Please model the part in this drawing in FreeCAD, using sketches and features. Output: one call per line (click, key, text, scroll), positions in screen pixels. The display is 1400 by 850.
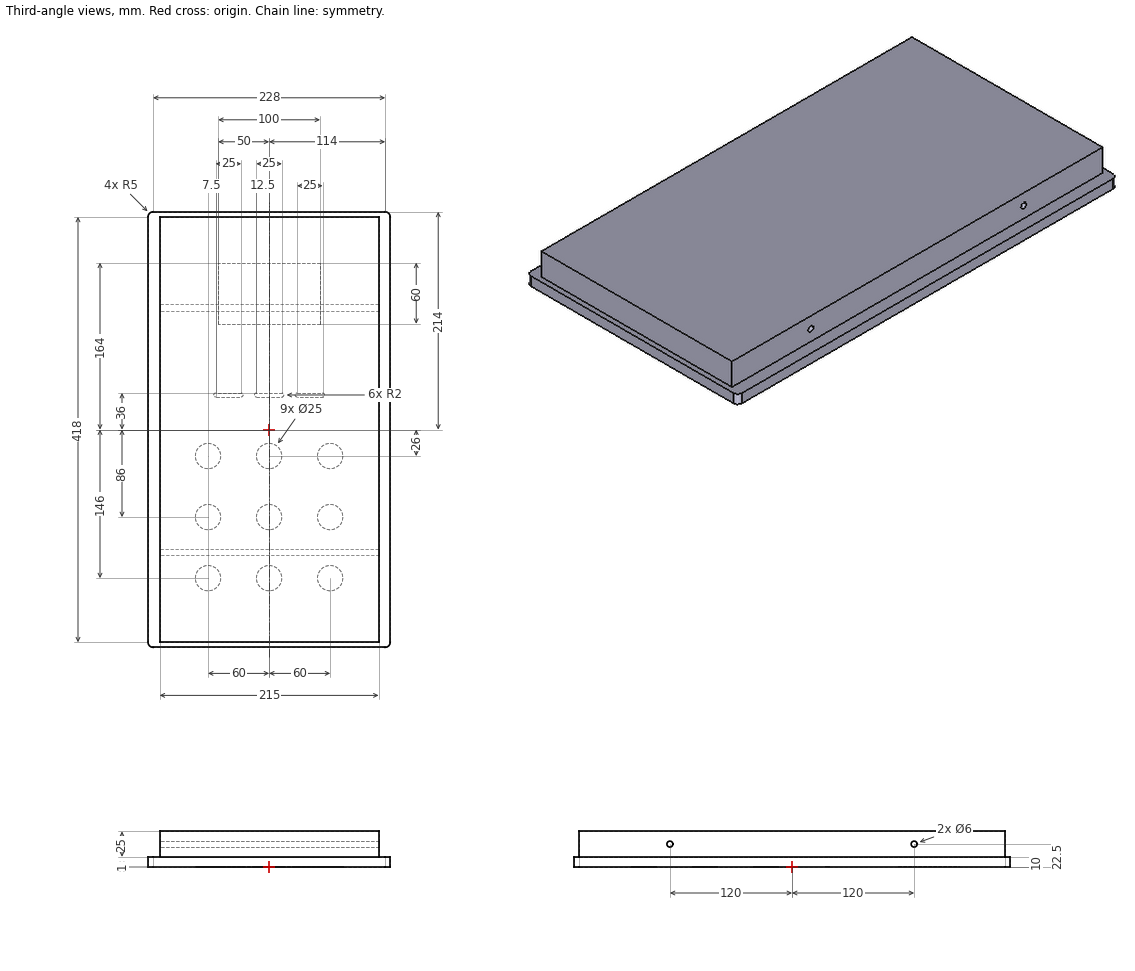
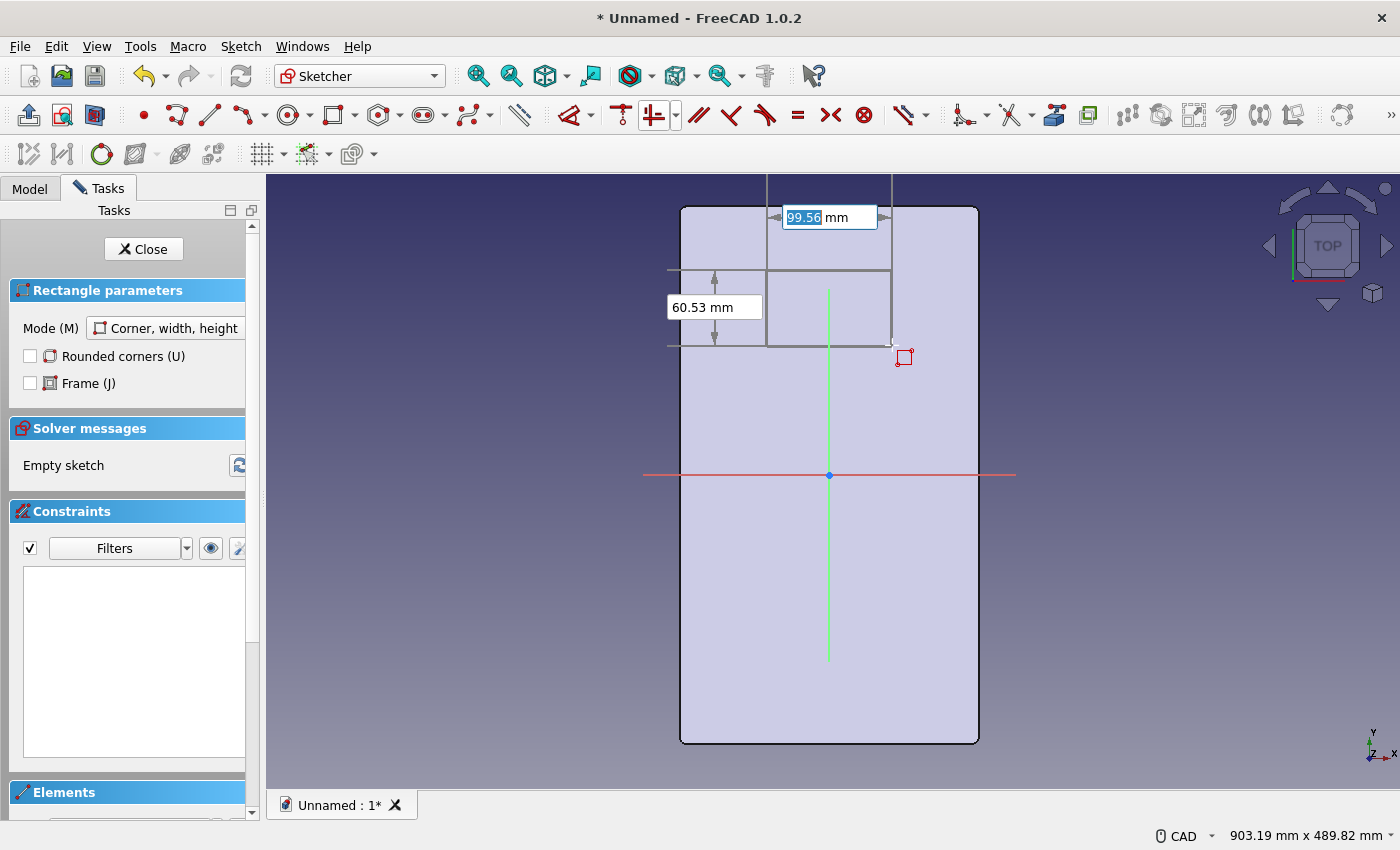
text(100)
key(Tab)
text(60)
key(Return)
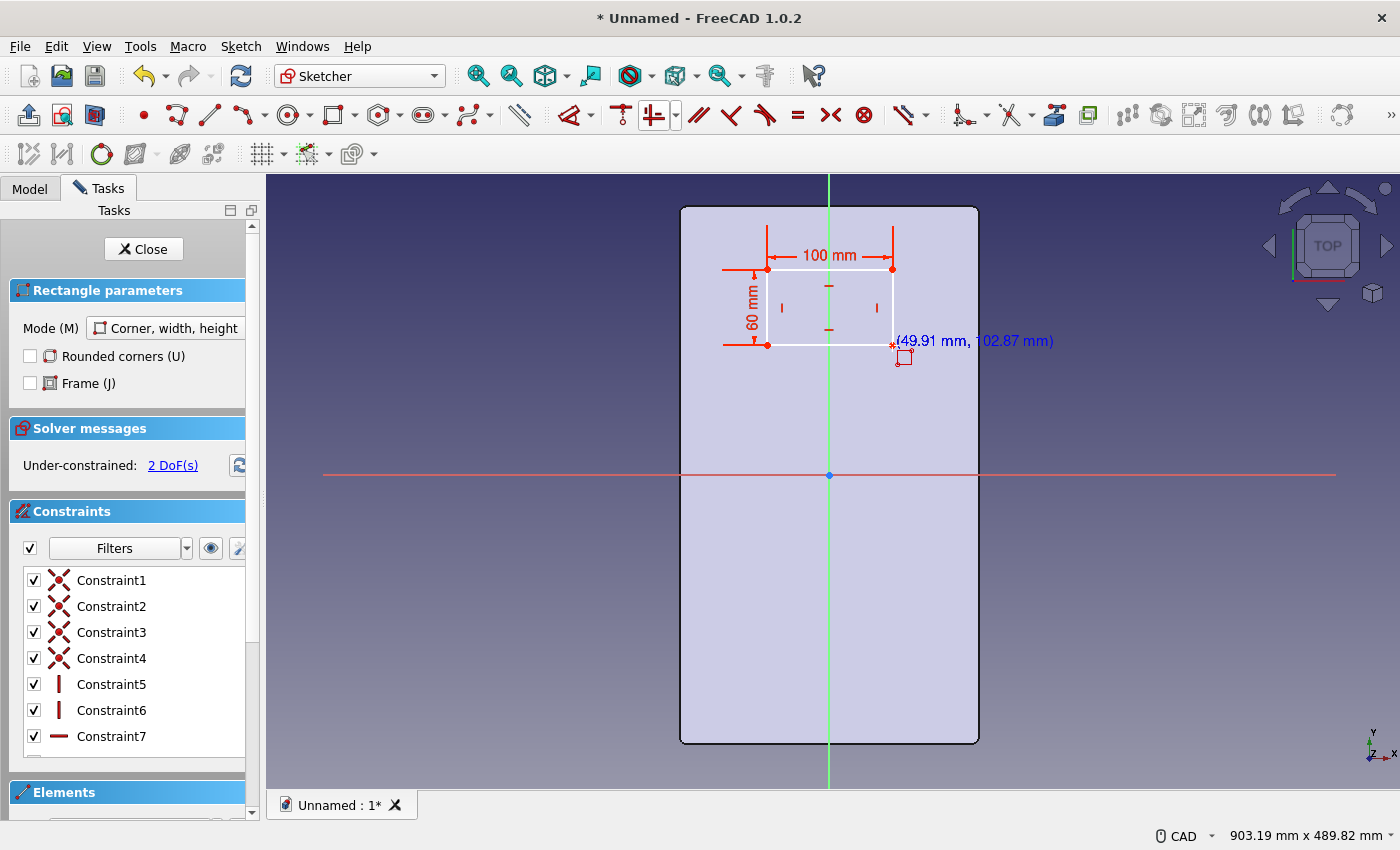
key(g)
key(s)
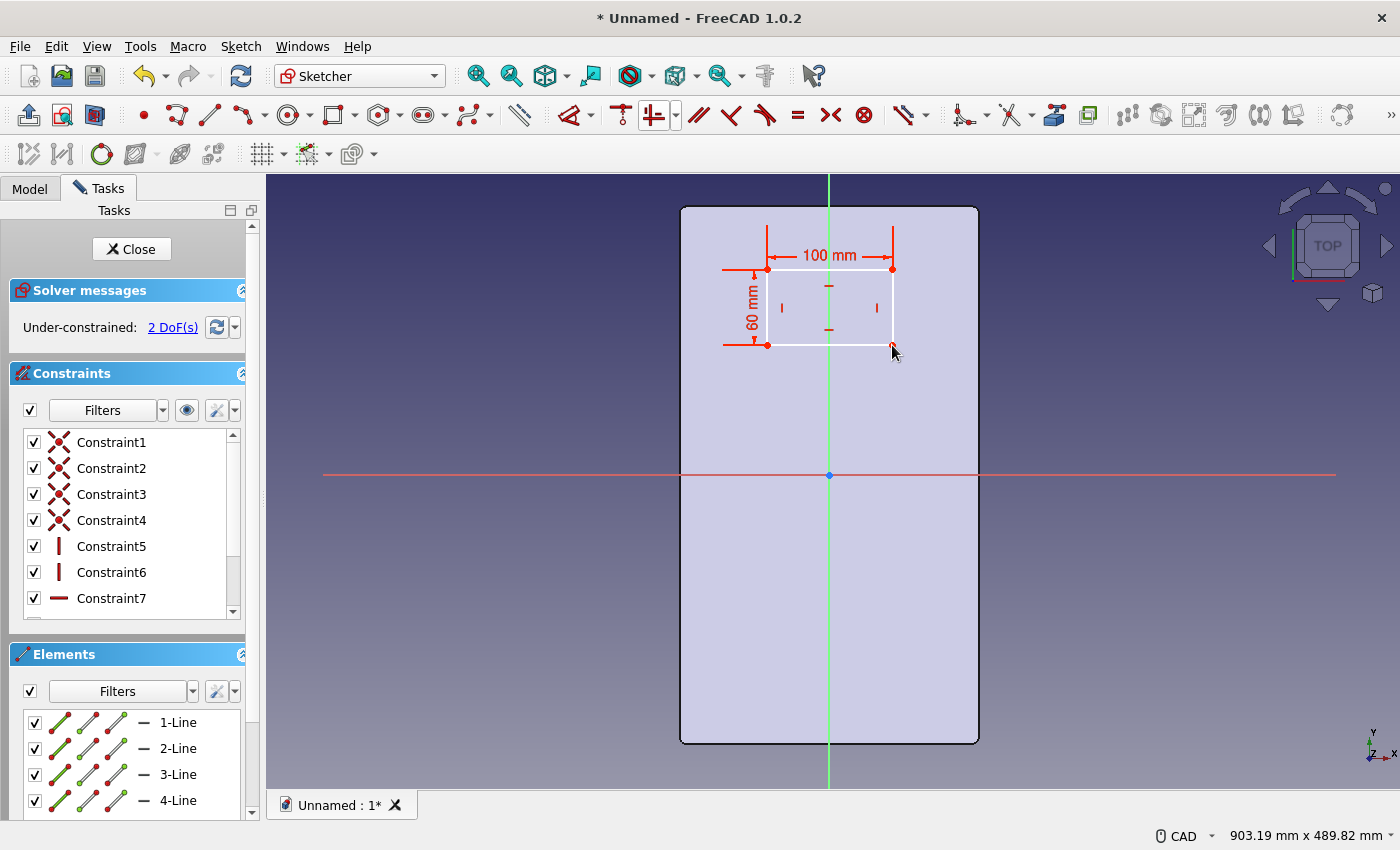
scroll(814, 432, up, 12)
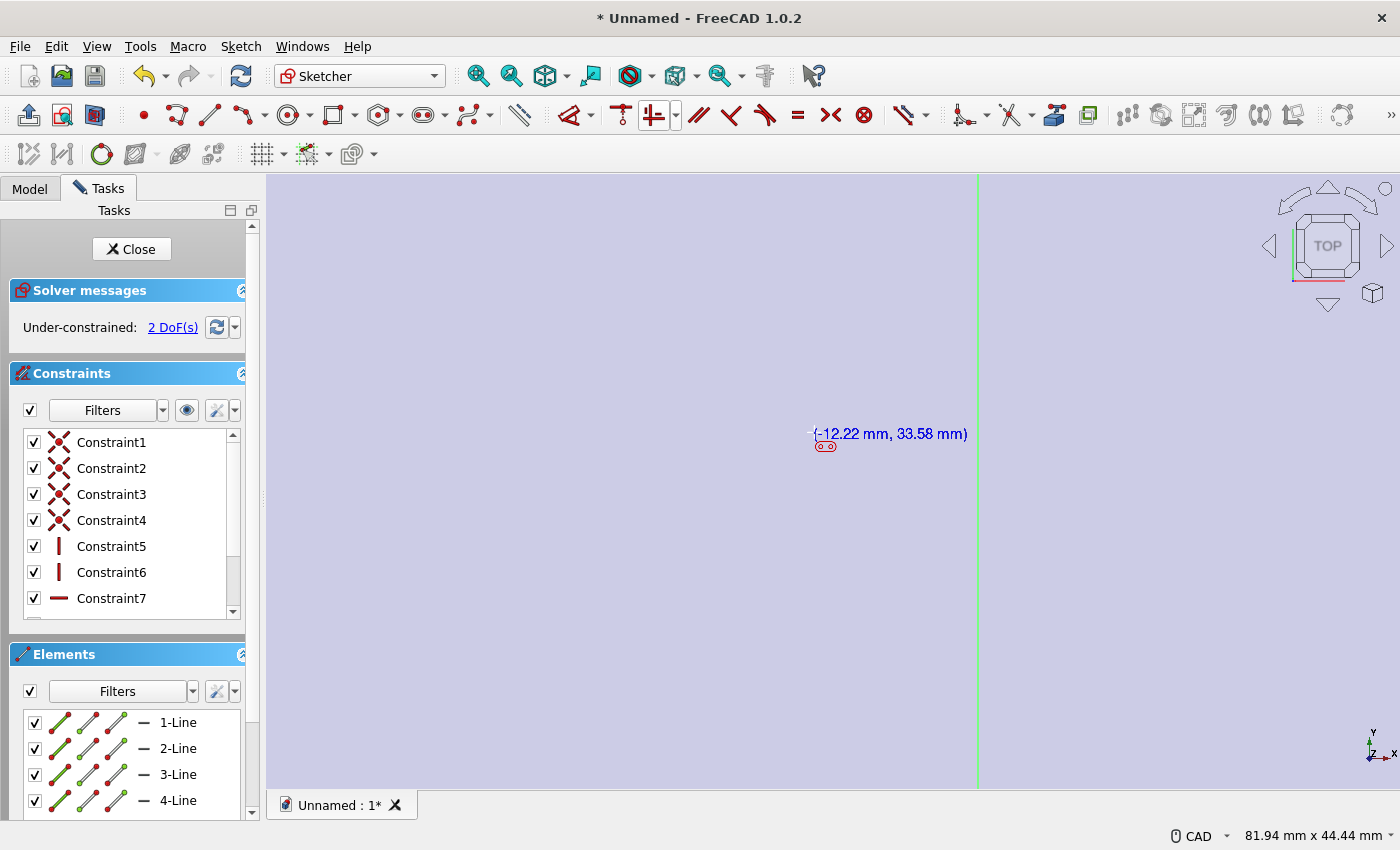
scroll(743, 443, down, 12)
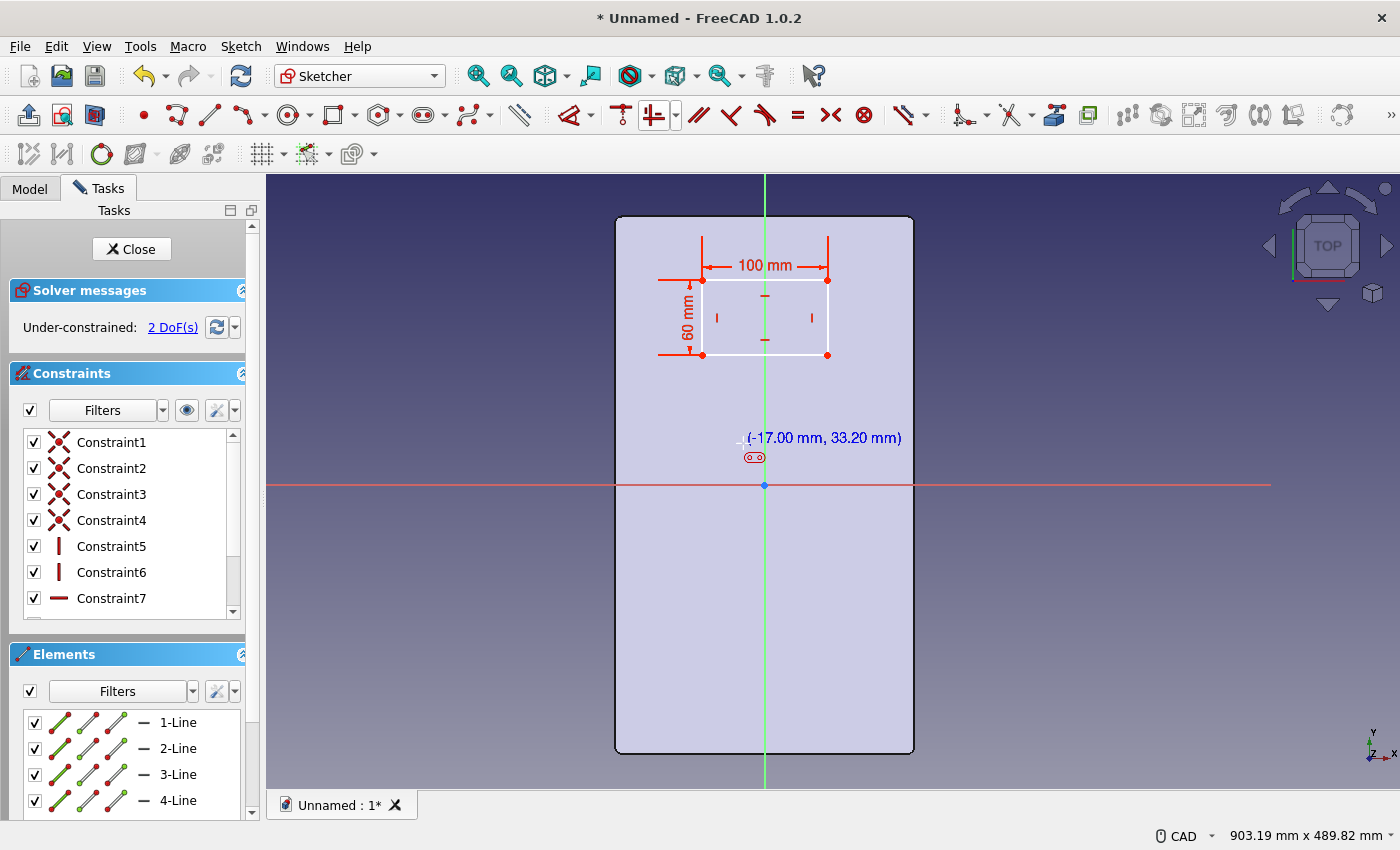
click(749, 442)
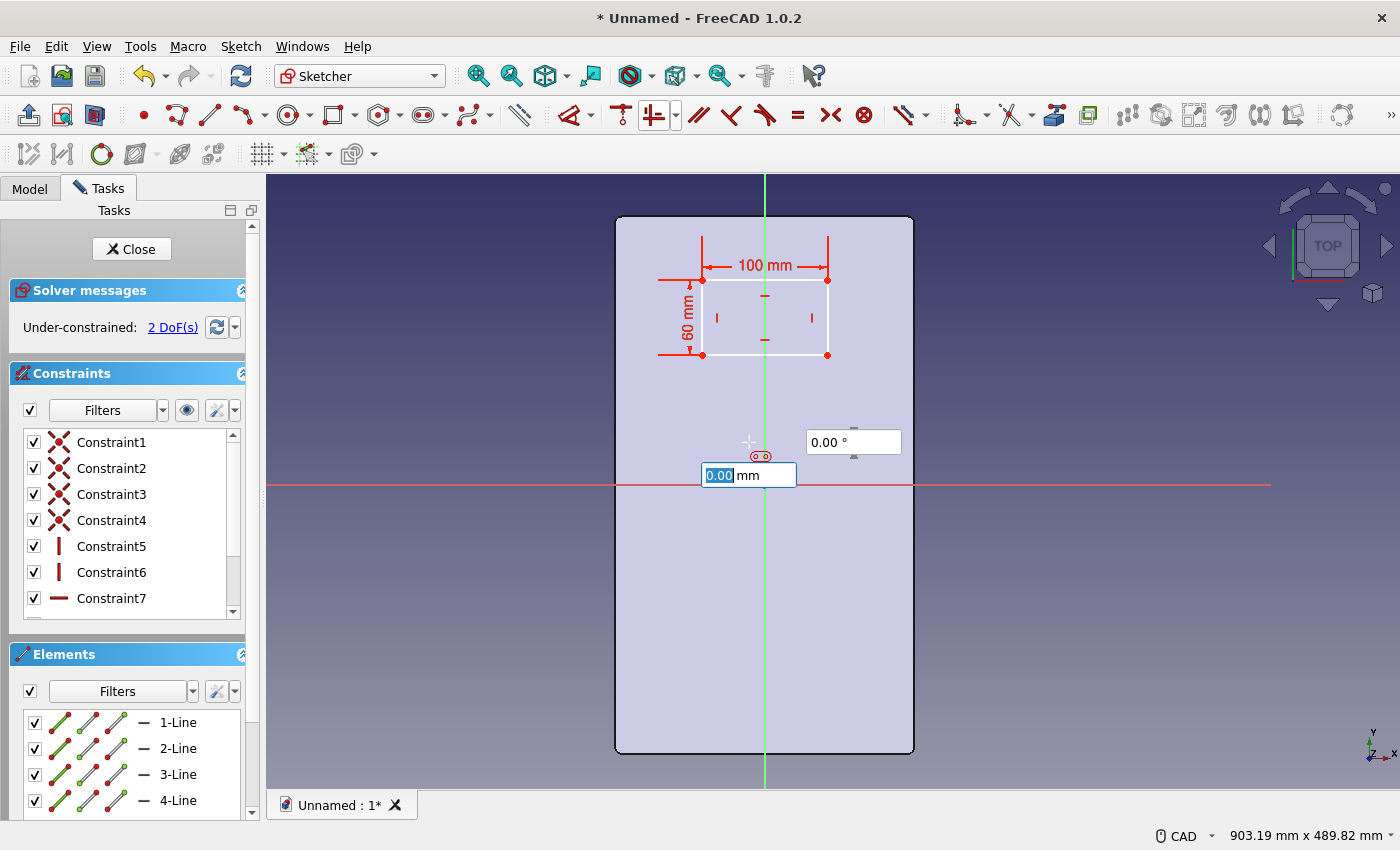
click(780, 442)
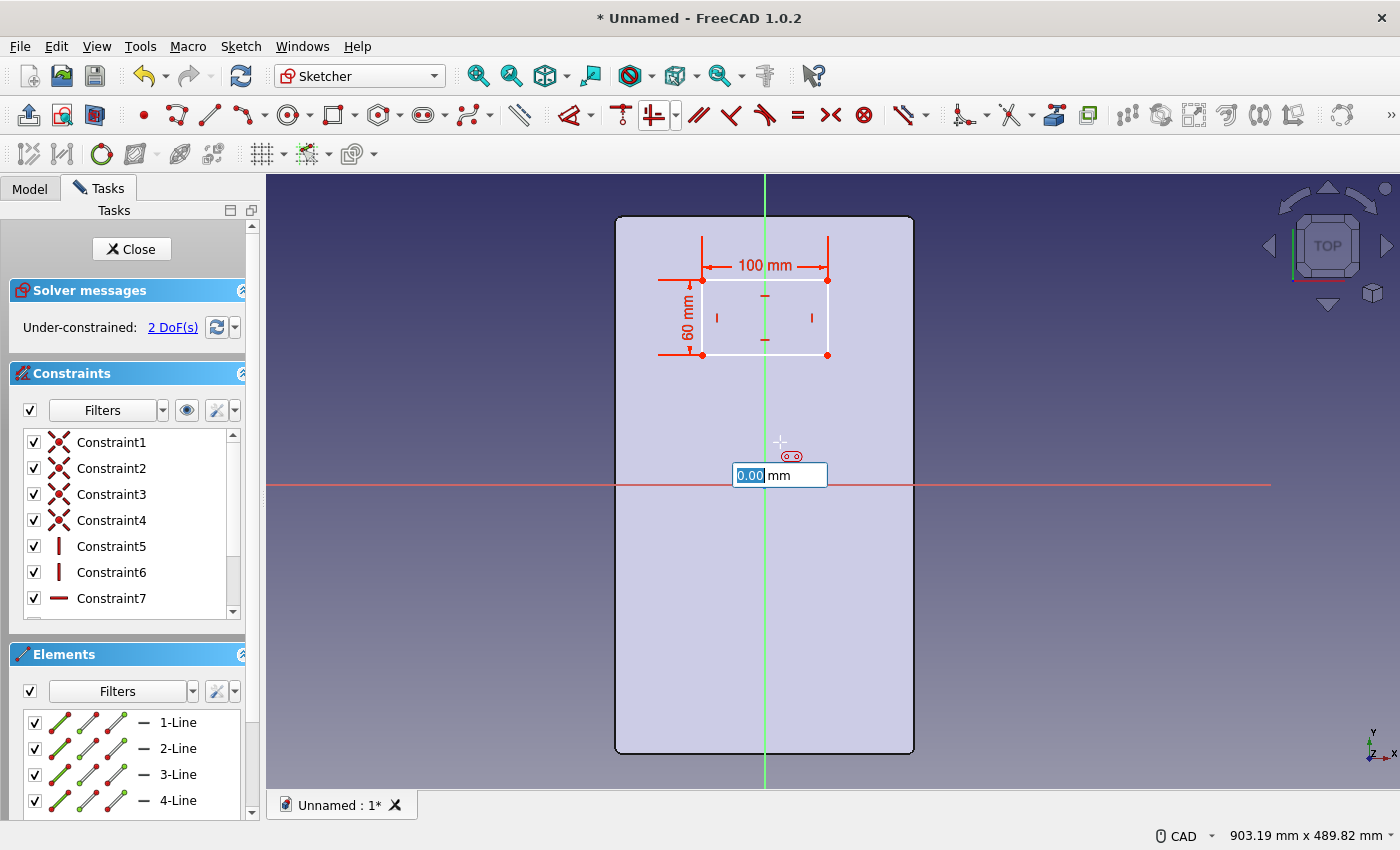
scroll(760, 440, up, 10)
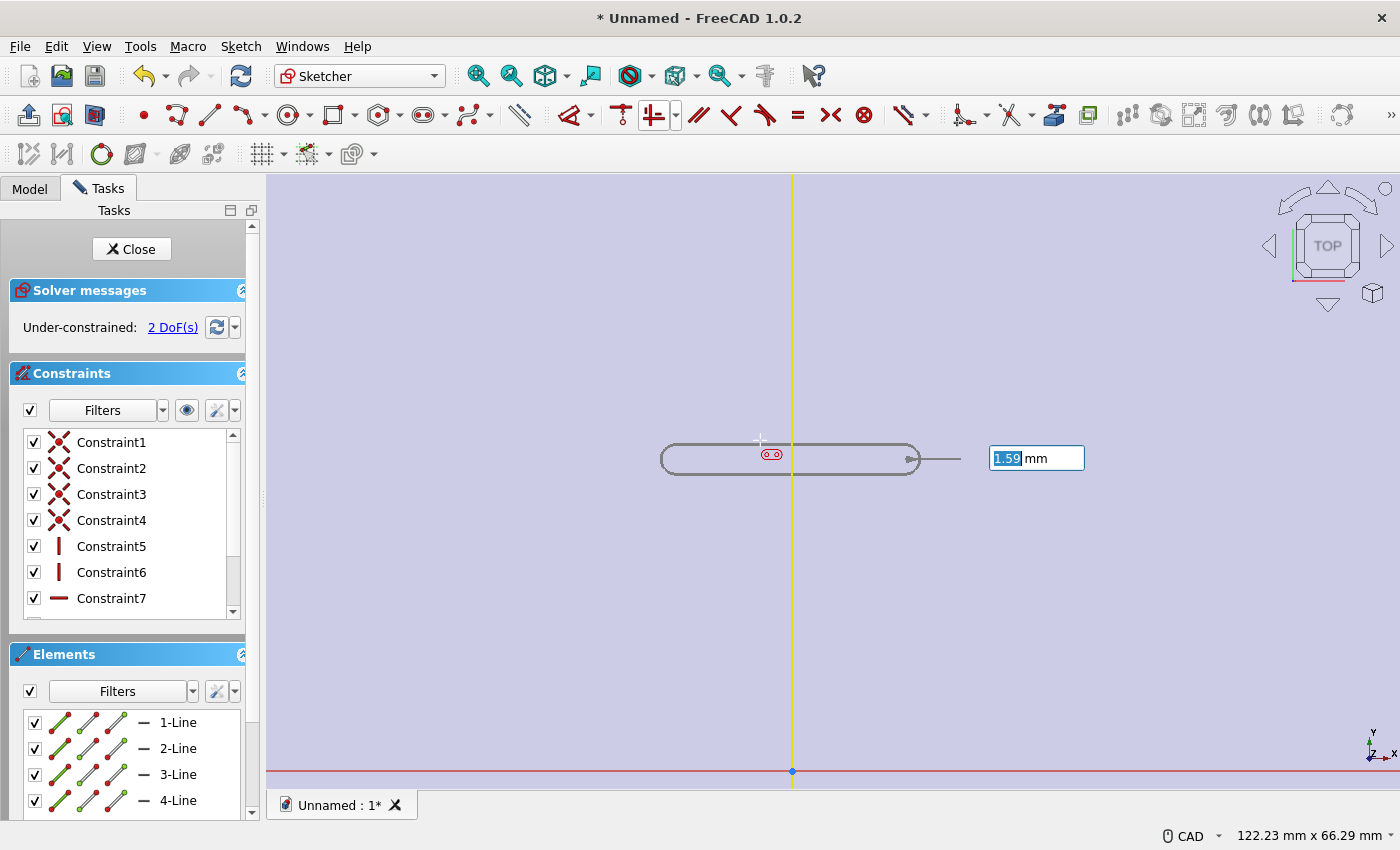
click(757, 437)